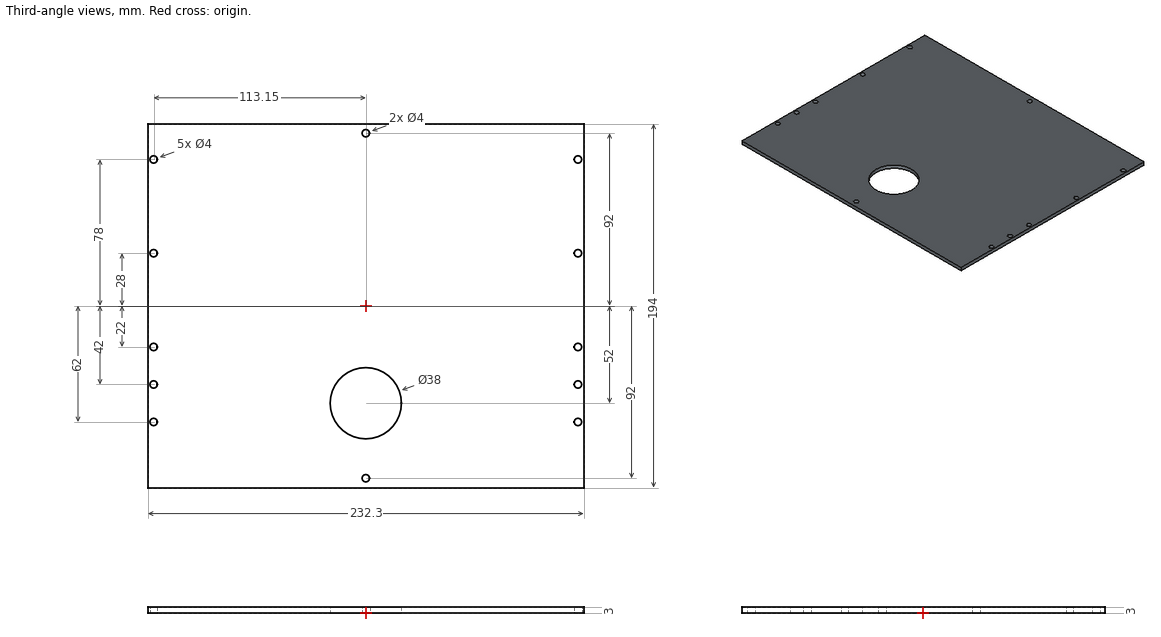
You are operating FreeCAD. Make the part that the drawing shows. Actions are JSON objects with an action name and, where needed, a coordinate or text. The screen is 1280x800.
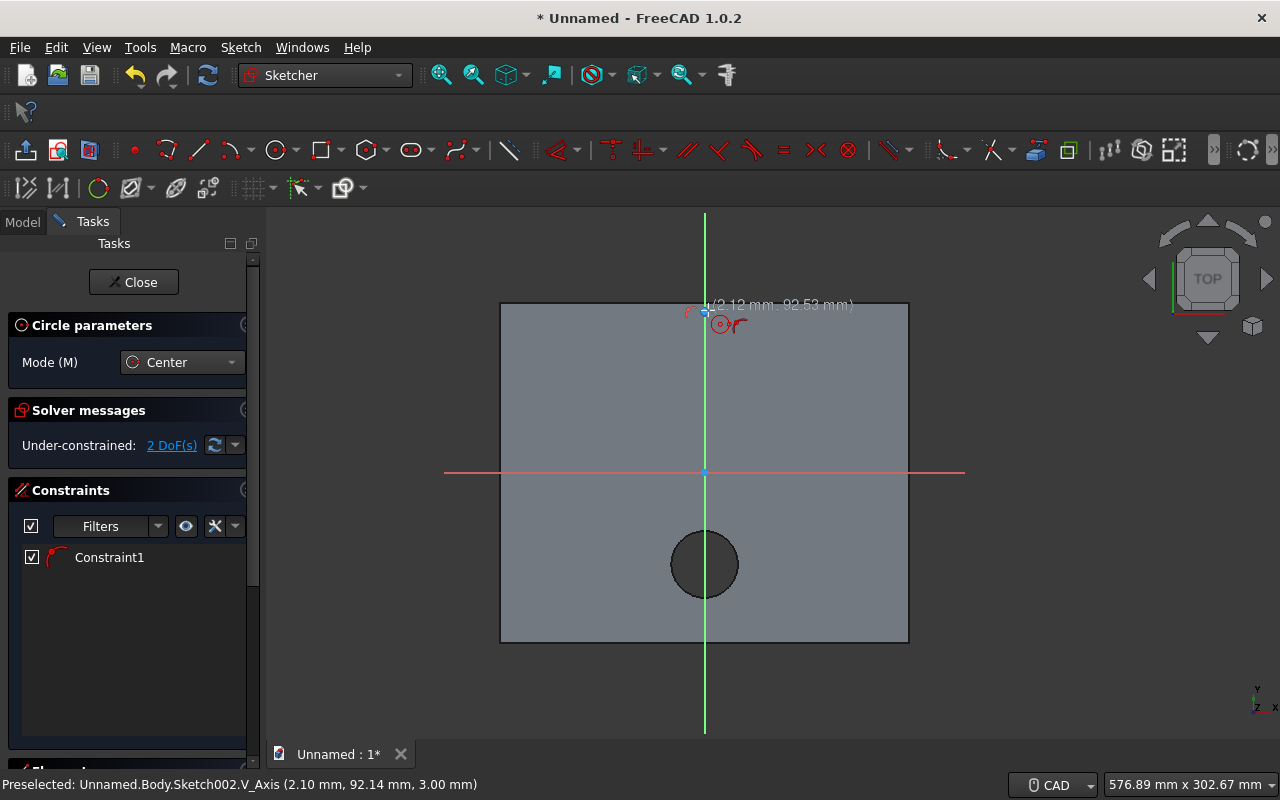
{"action": "scroll", "coordinate": [705, 635], "scroll_direction": "up", "scroll_amount": 10}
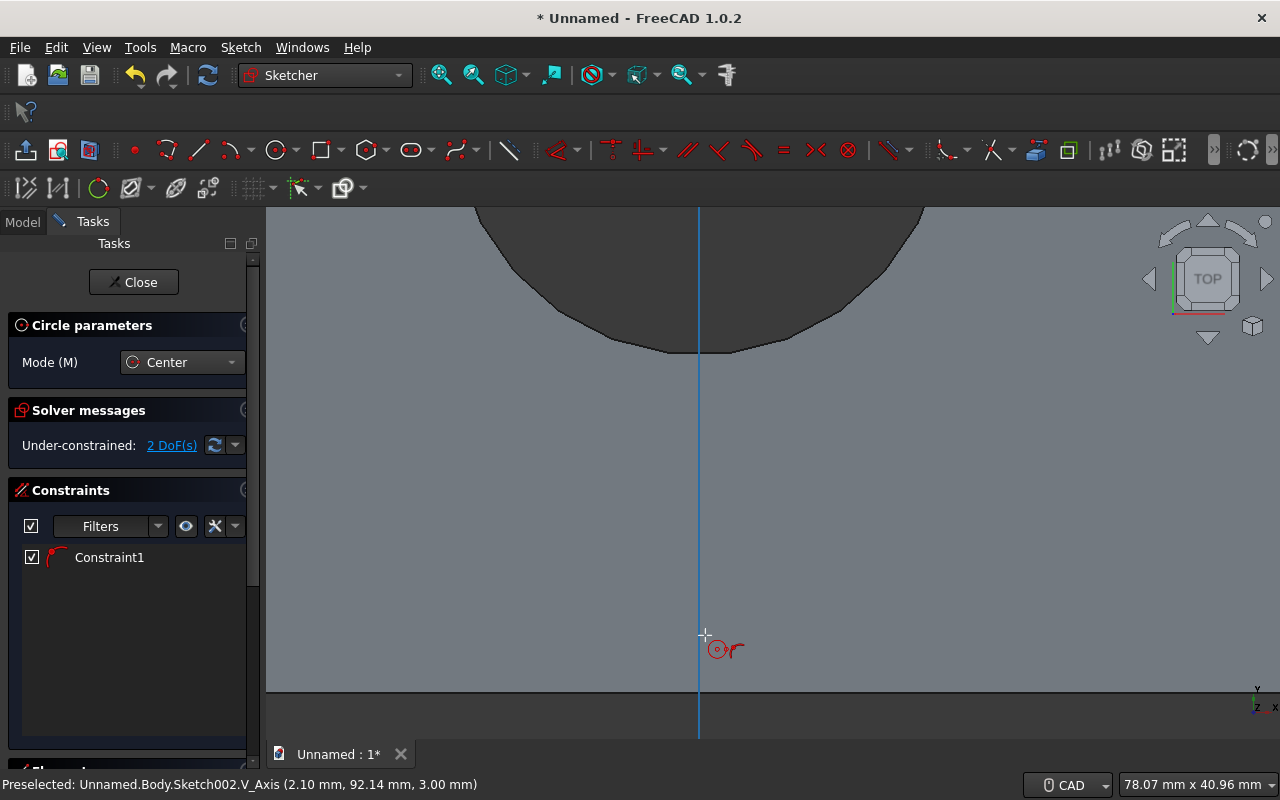
{"action": "scroll", "coordinate": [705, 636], "scroll_direction": "down", "scroll_amount": 10}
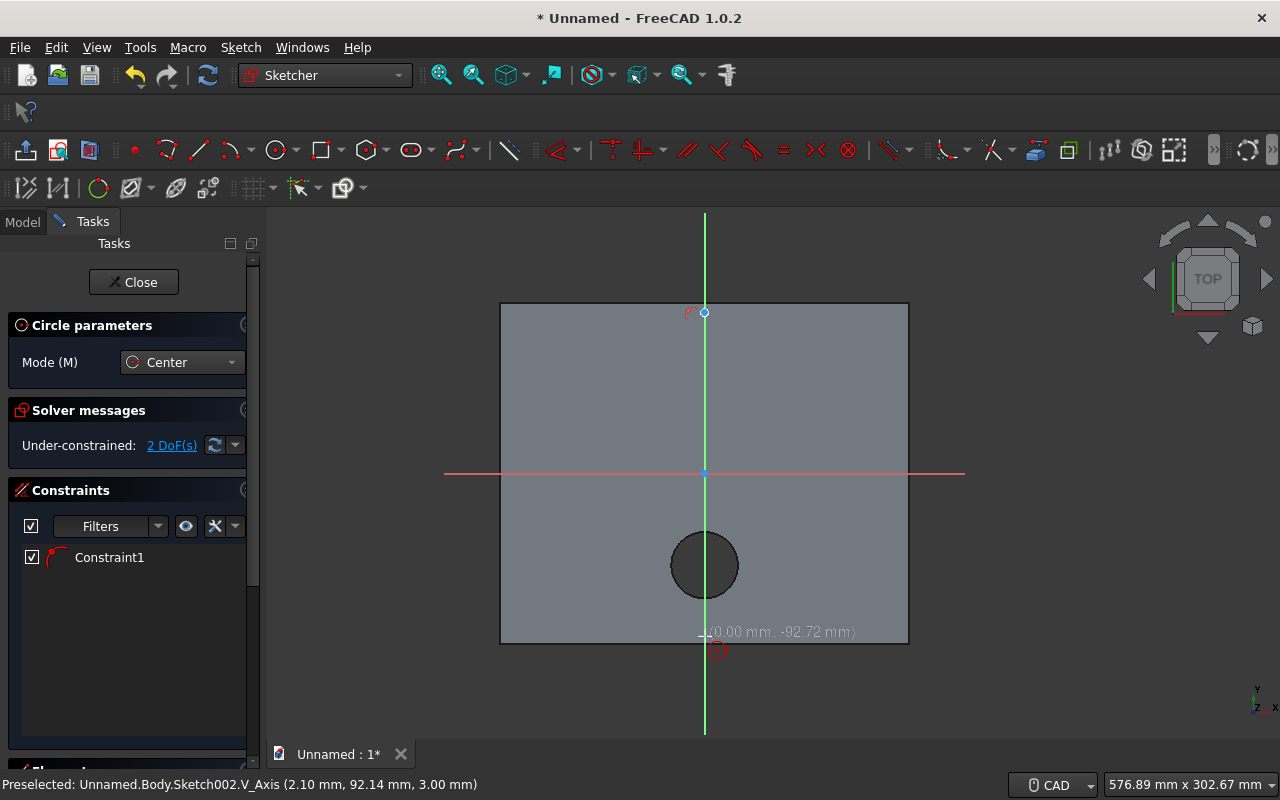
{"action": "left_click", "coordinate": [705, 636]}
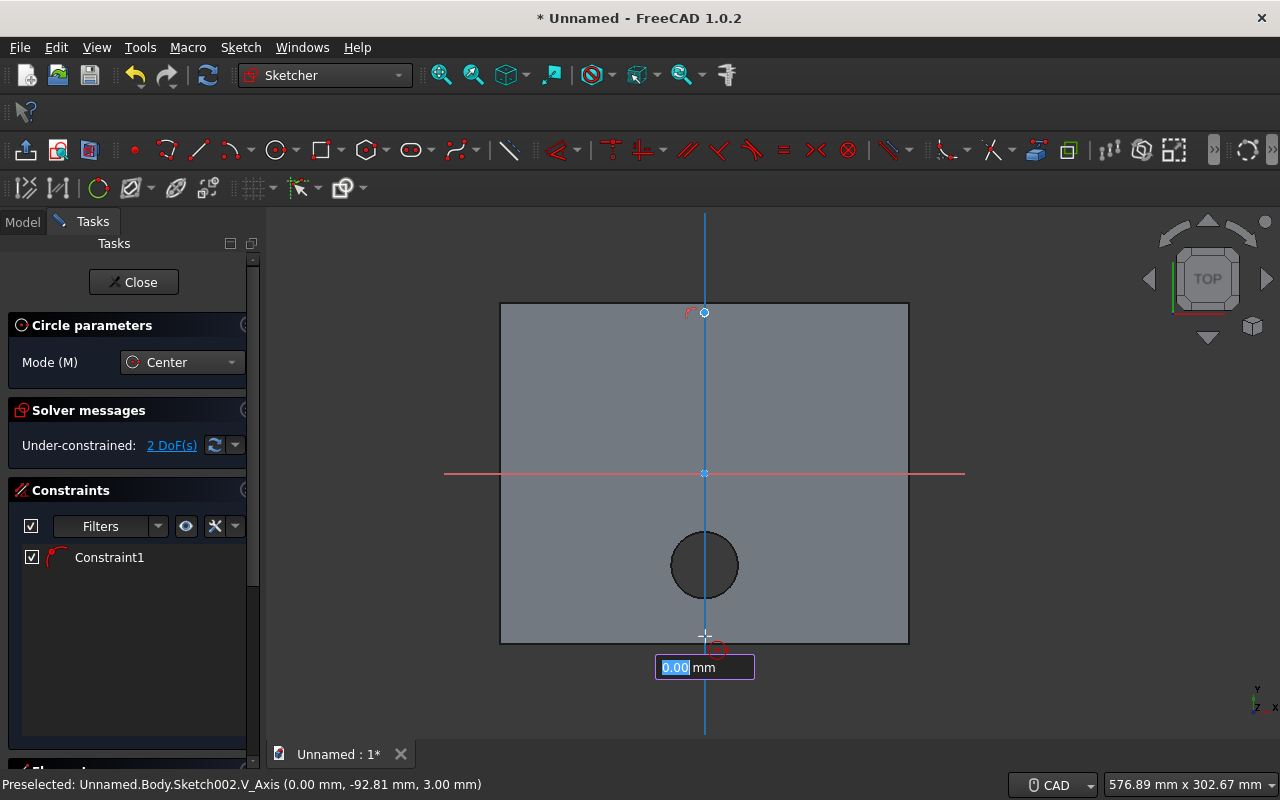
{"action": "scroll", "coordinate": [708, 634], "scroll_direction": "up", "scroll_amount": 8}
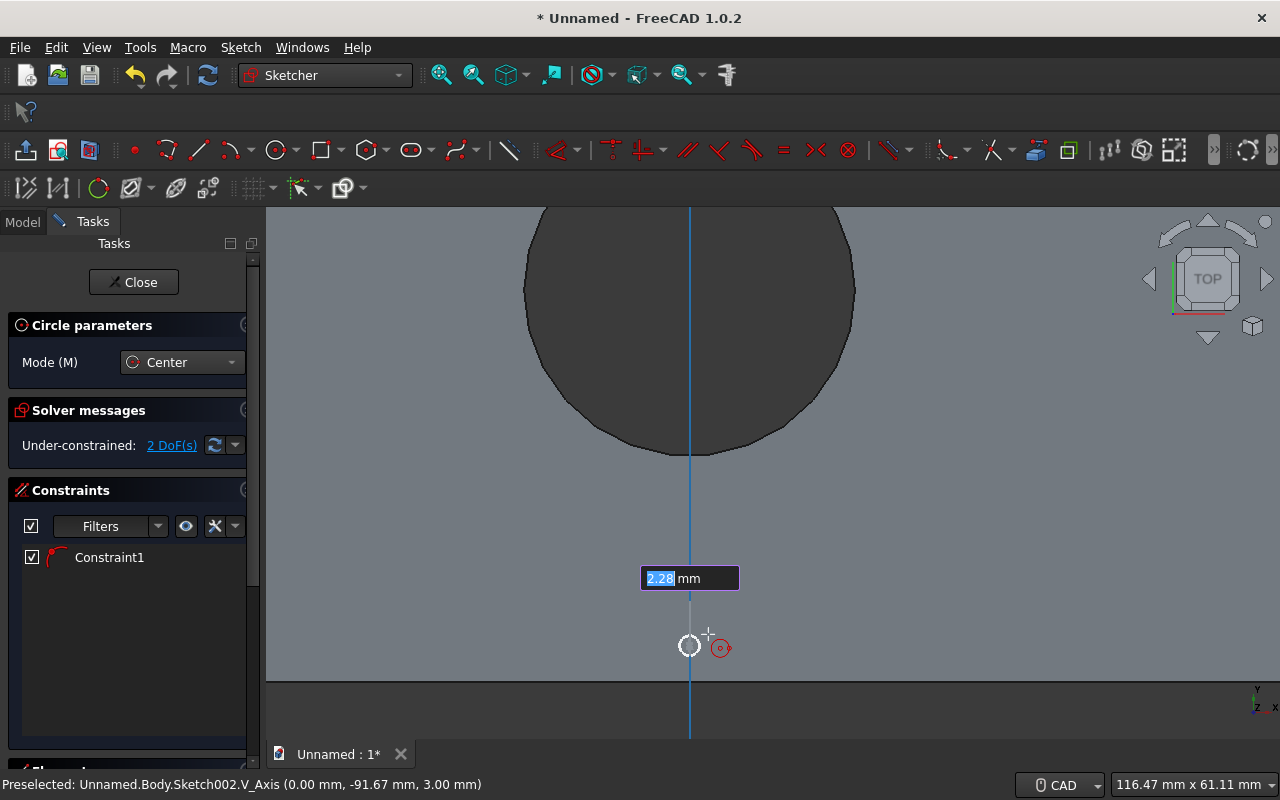
{"action": "left_click", "coordinate": [706, 633]}
{"action": "key", "text": "Escape"}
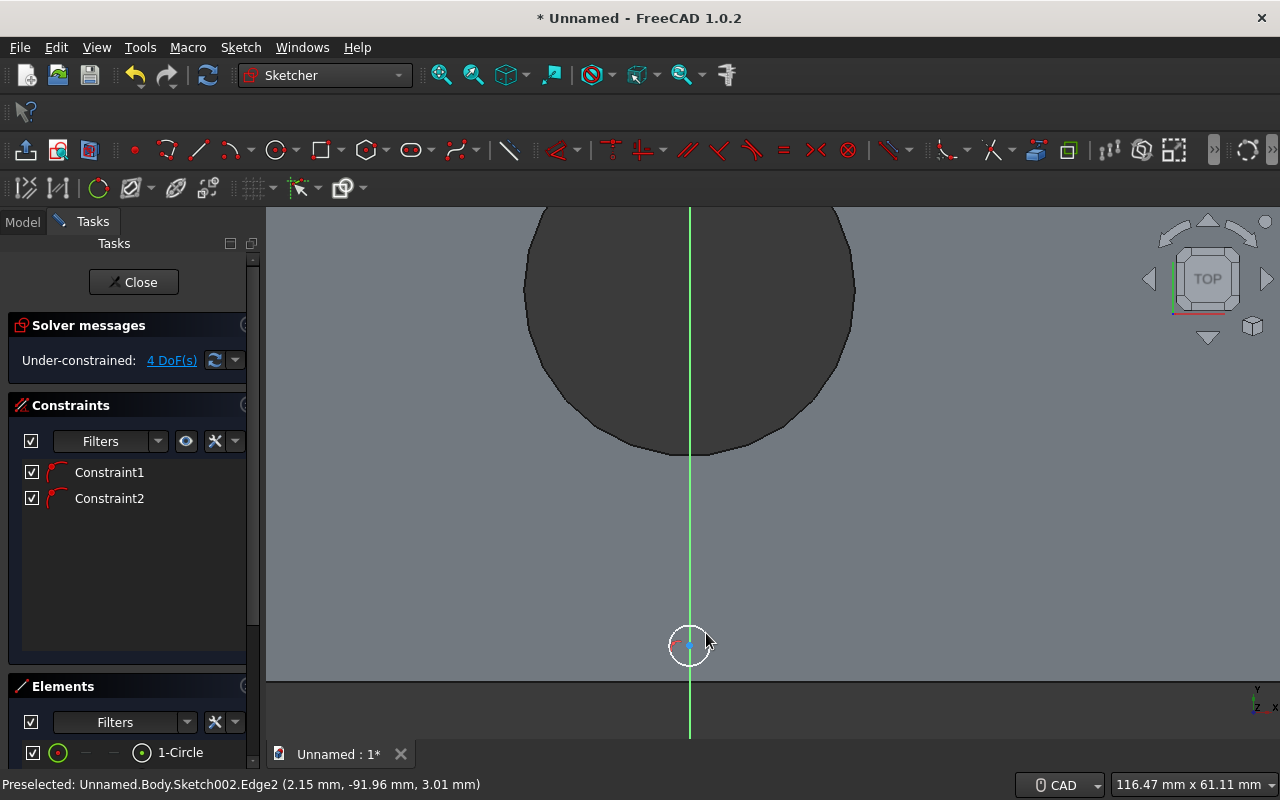
{"action": "scroll", "coordinate": [708, 634], "scroll_direction": "down", "scroll_amount": 8}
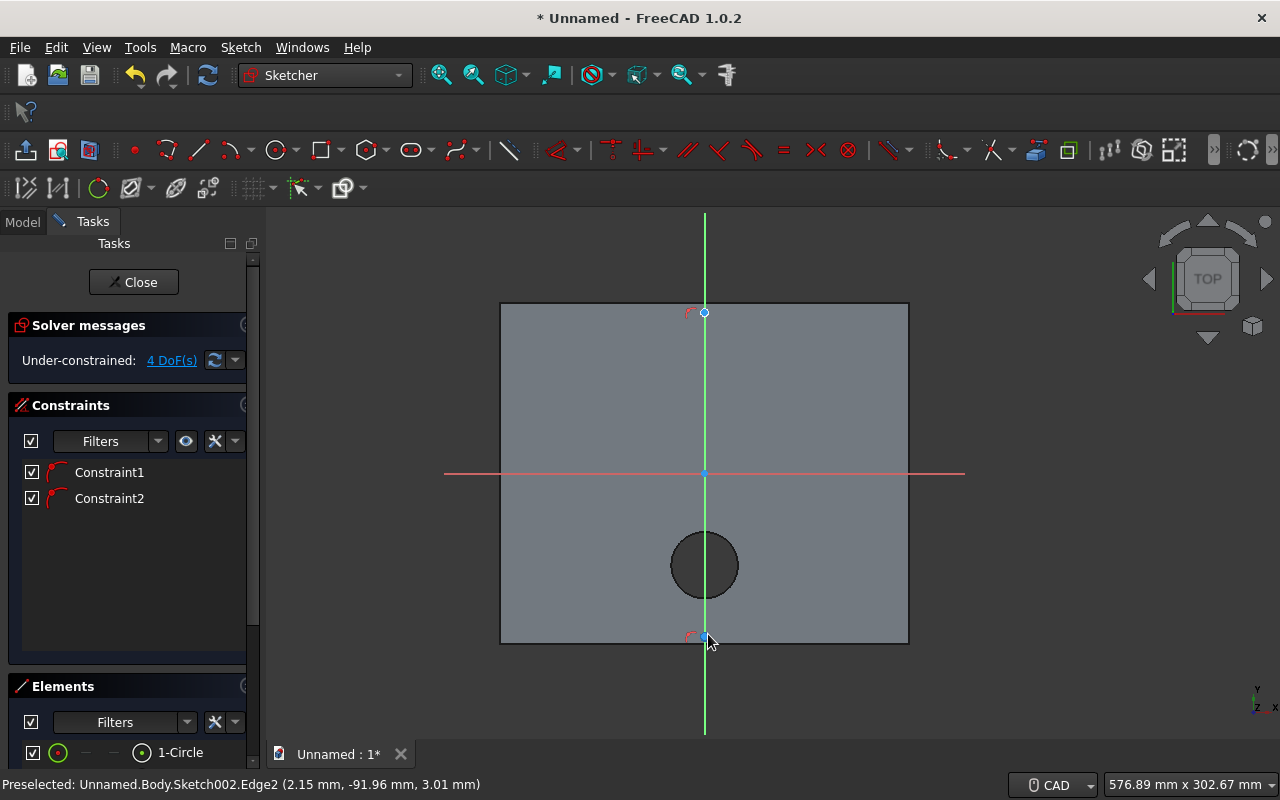
{"action": "scroll", "coordinate": [707, 310], "scroll_direction": "up", "scroll_amount": 9}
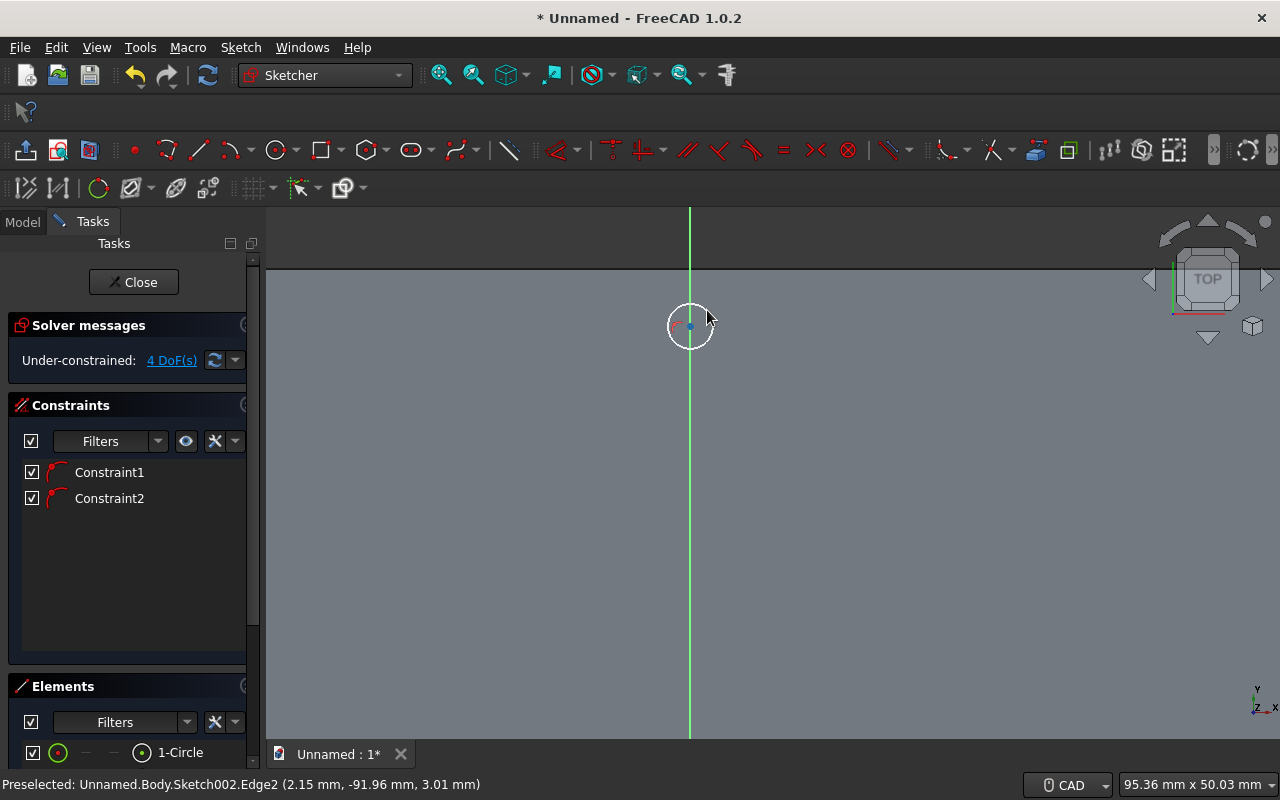
{"action": "left_click", "coordinate": [706, 310]}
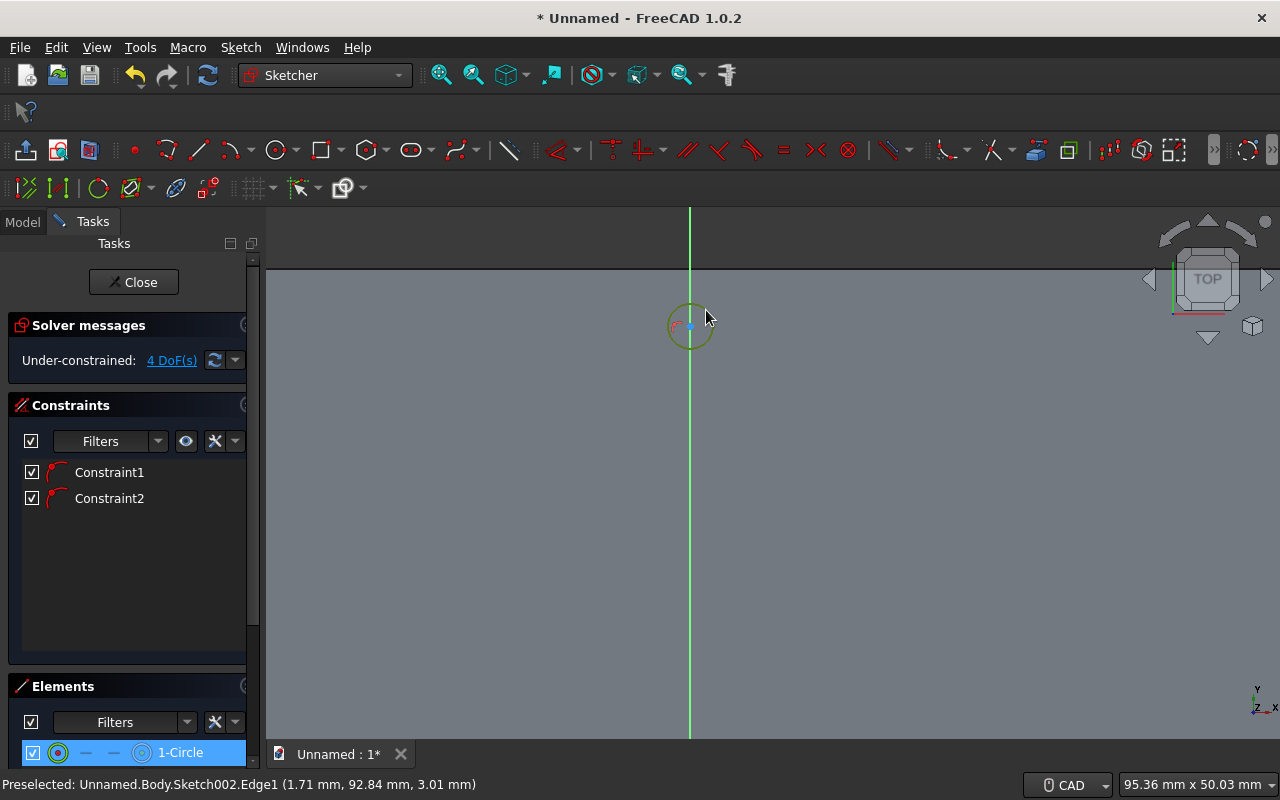
{"action": "scroll", "coordinate": [707, 309], "scroll_direction": "down", "scroll_amount": 9}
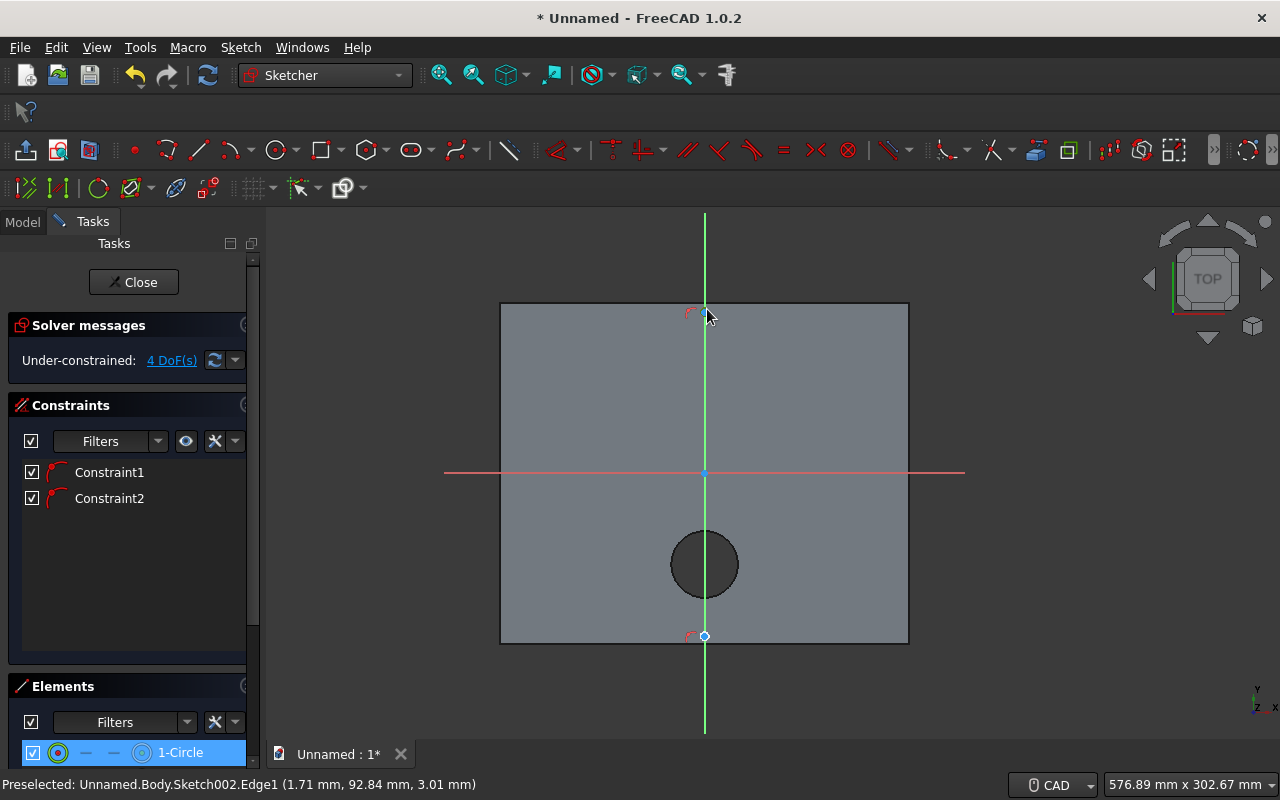
{"action": "scroll", "coordinate": [707, 633], "scroll_direction": "up", "scroll_amount": 8}